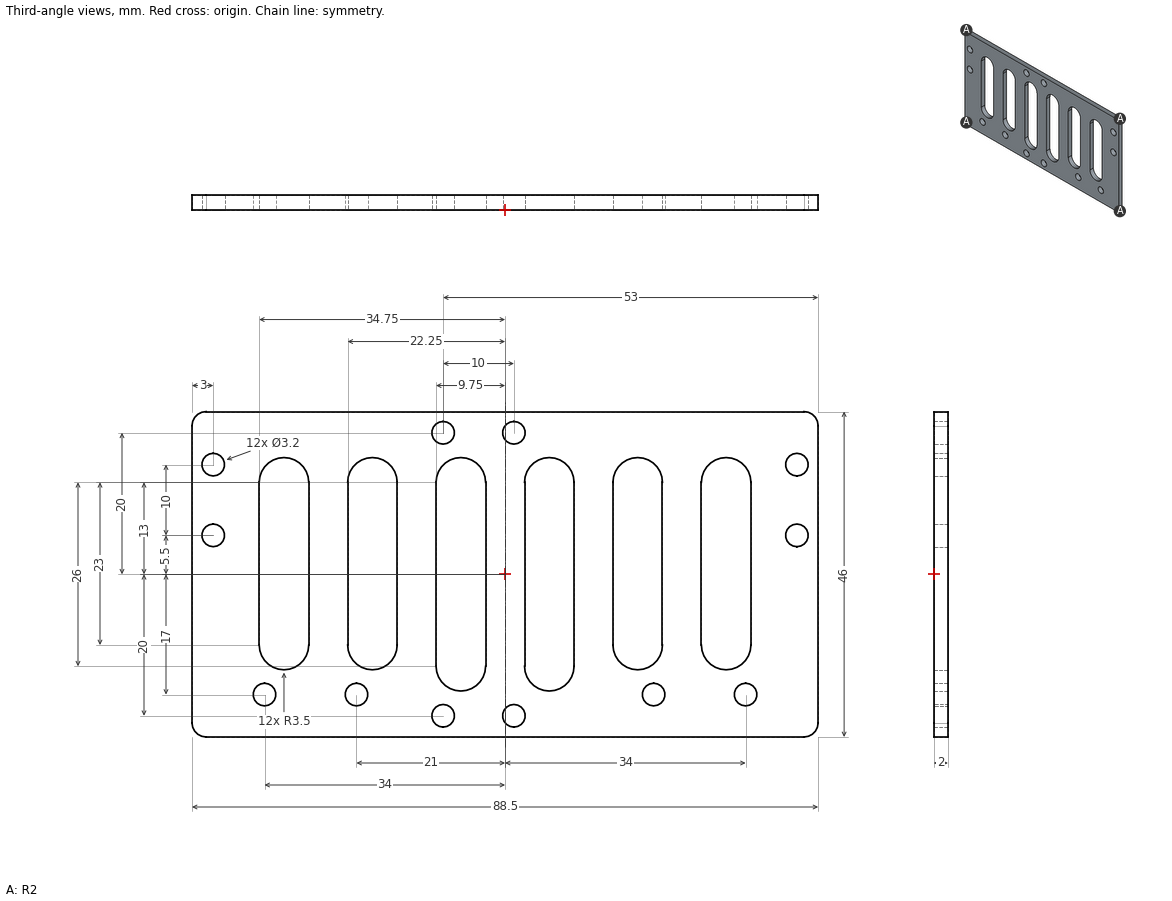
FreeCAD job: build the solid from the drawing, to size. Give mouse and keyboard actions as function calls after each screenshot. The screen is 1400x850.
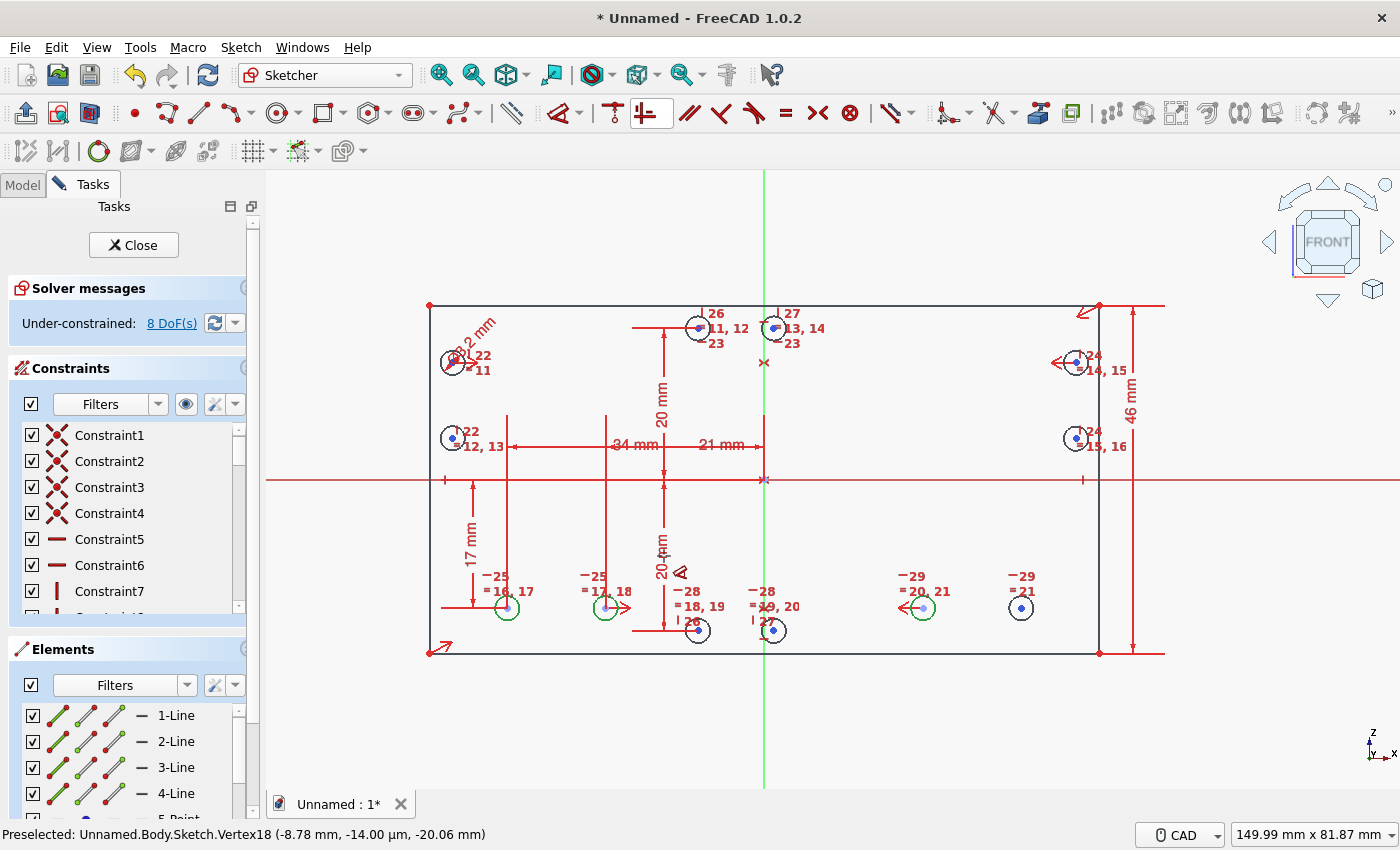
click(1021, 608)
click(893, 446)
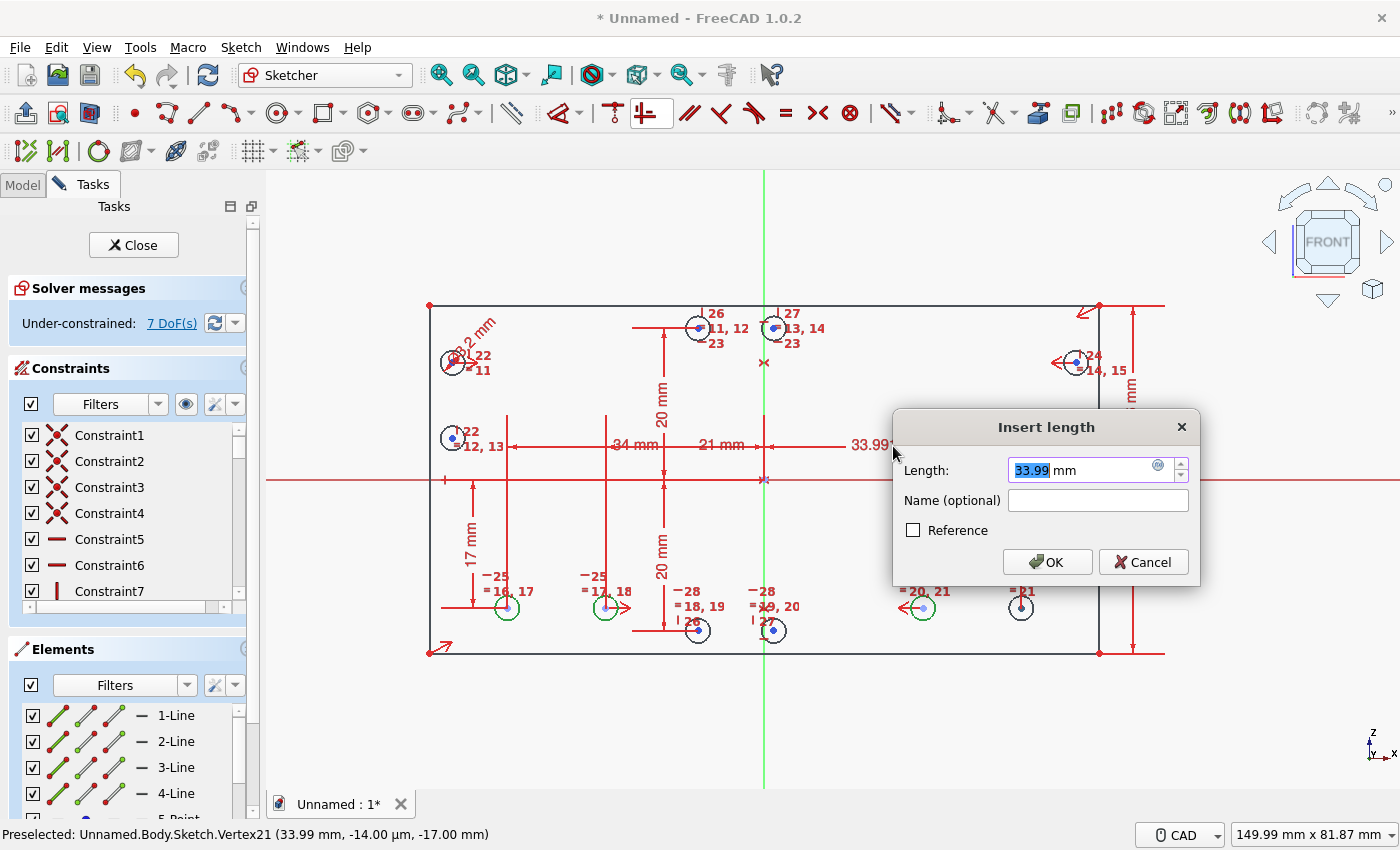
text(34)
key(Return)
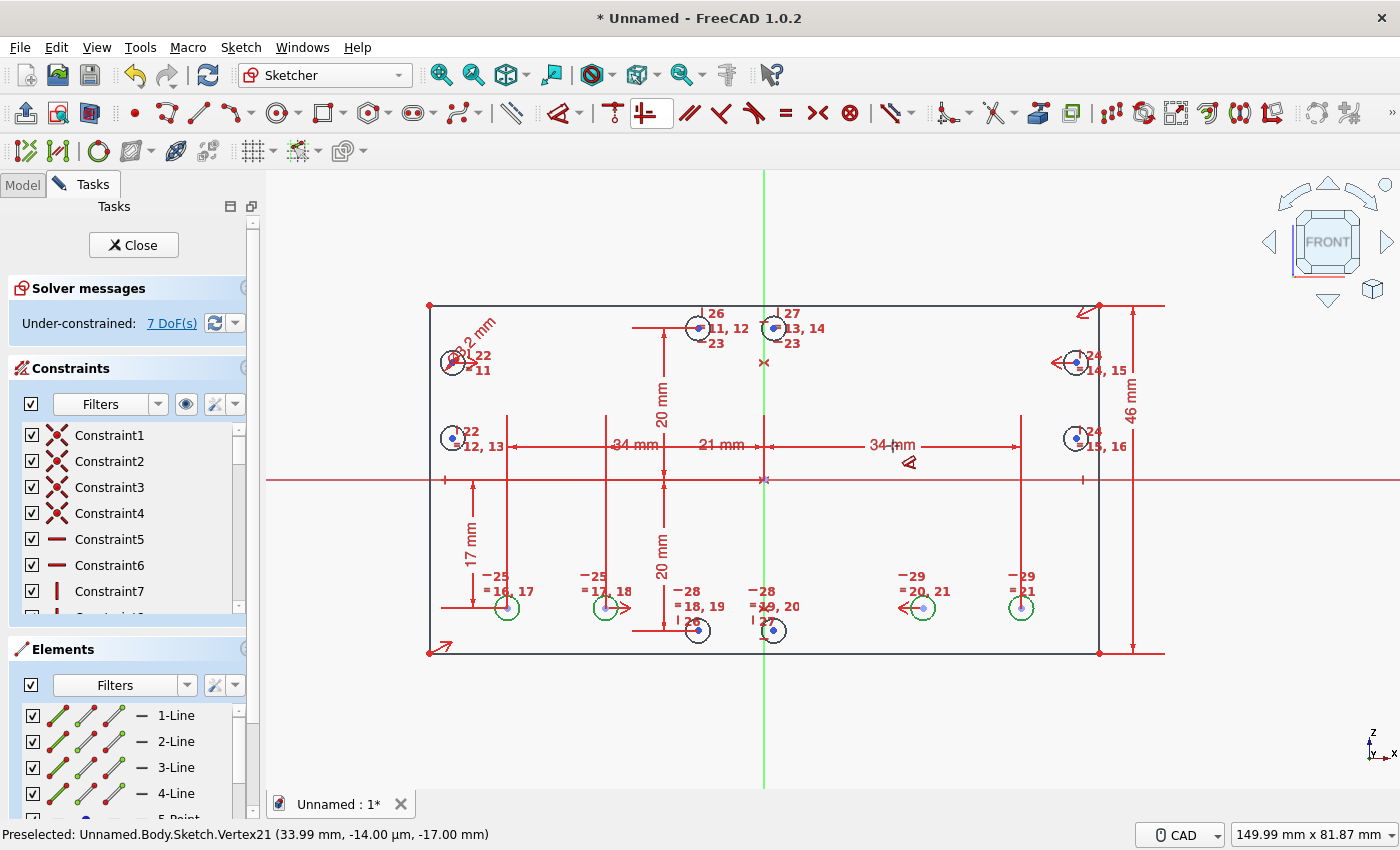
scroll(430, 306, up, 3)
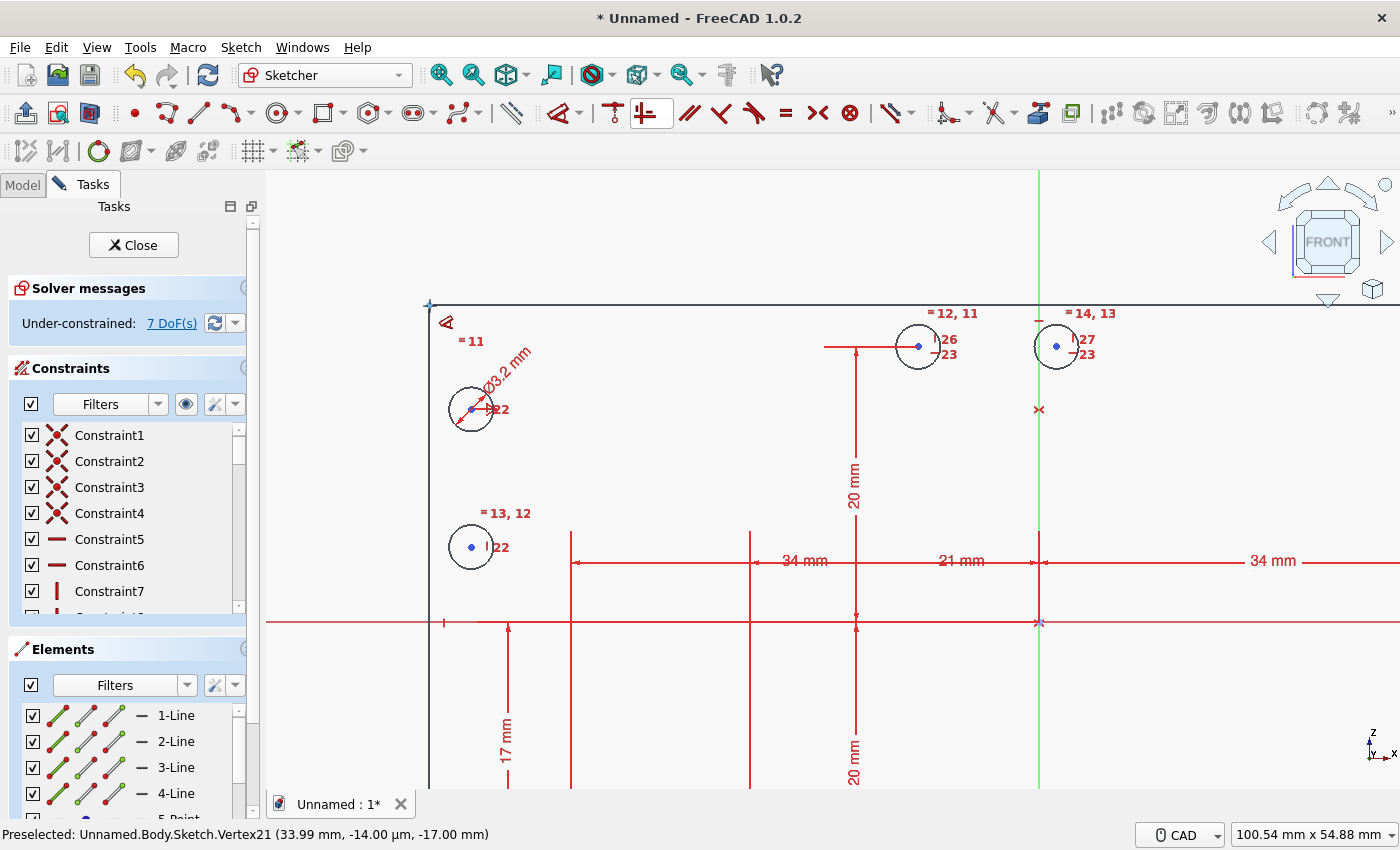
click(429, 305)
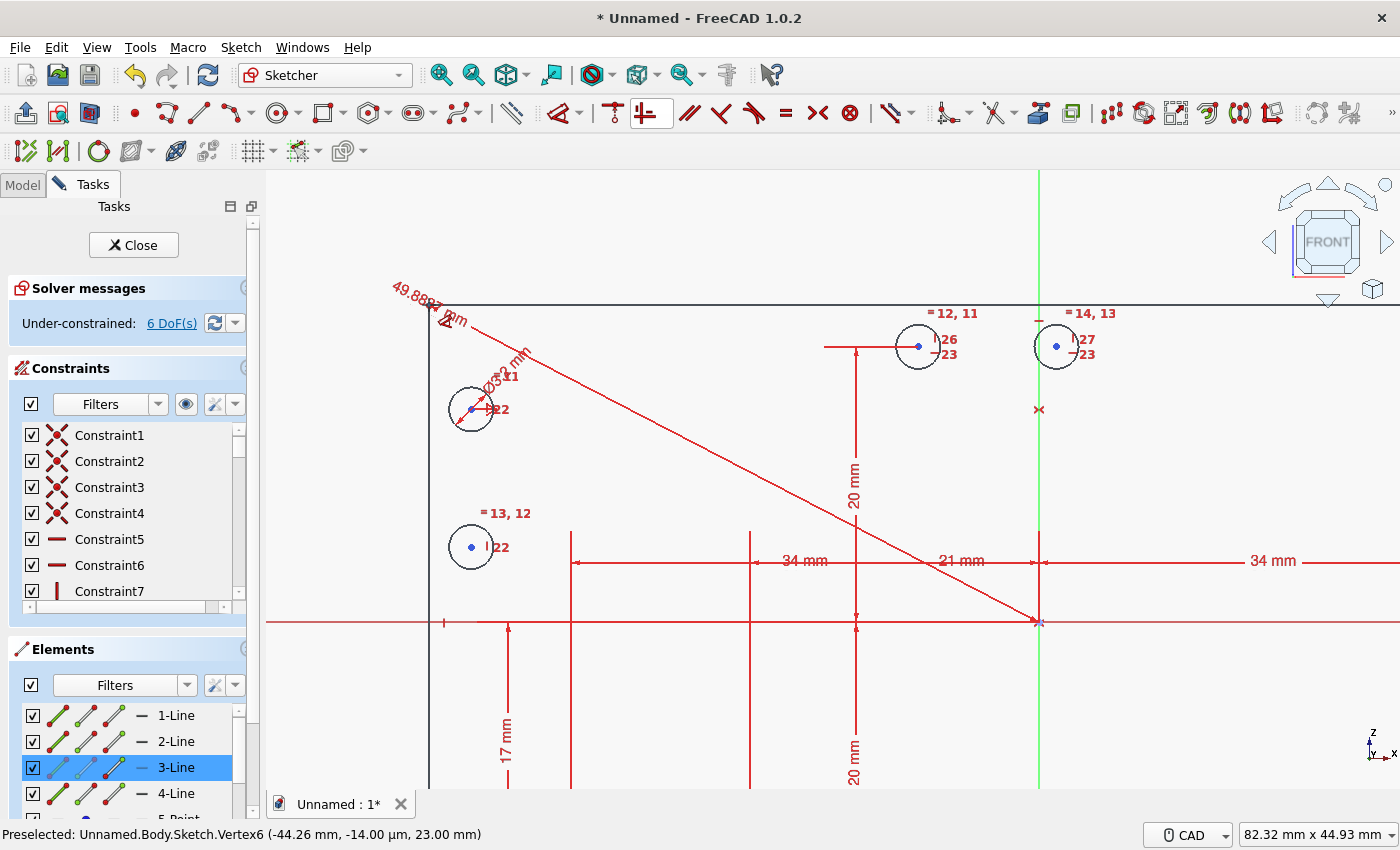
click(471, 409)
click(450, 271)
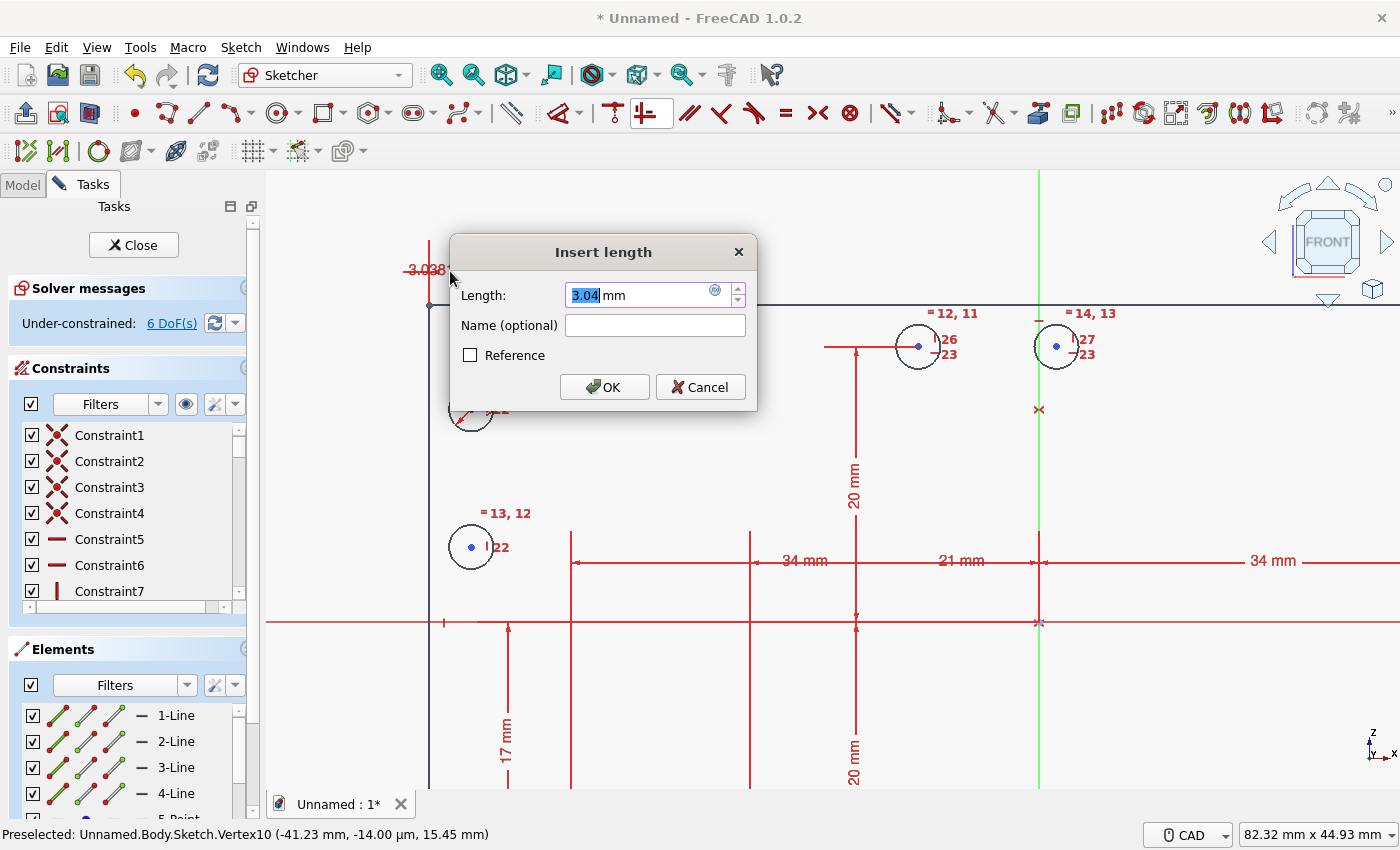
text(3)
key(Return)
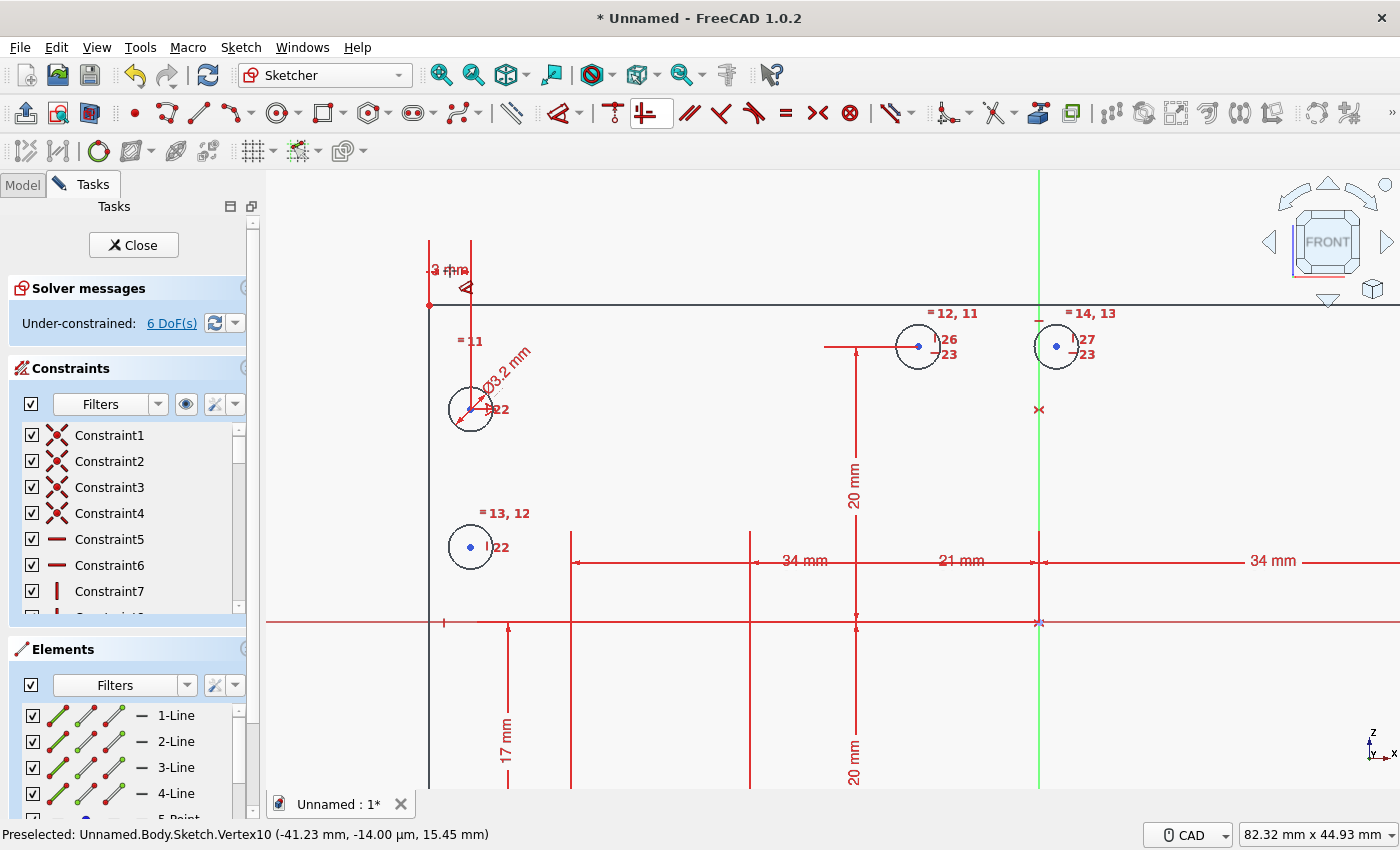
click(471, 547)
click(1073, 585)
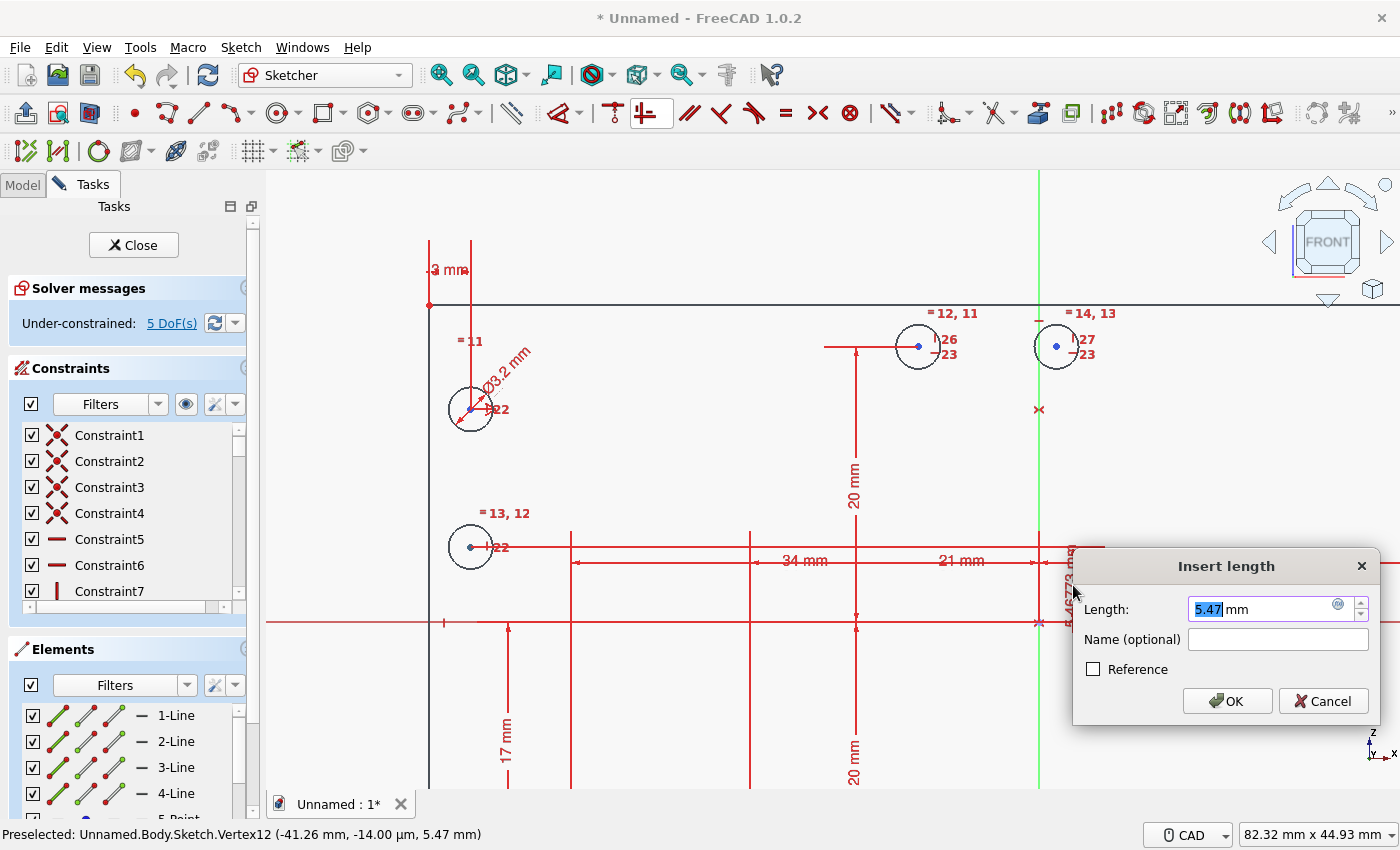
text(5.5)
key(Return)